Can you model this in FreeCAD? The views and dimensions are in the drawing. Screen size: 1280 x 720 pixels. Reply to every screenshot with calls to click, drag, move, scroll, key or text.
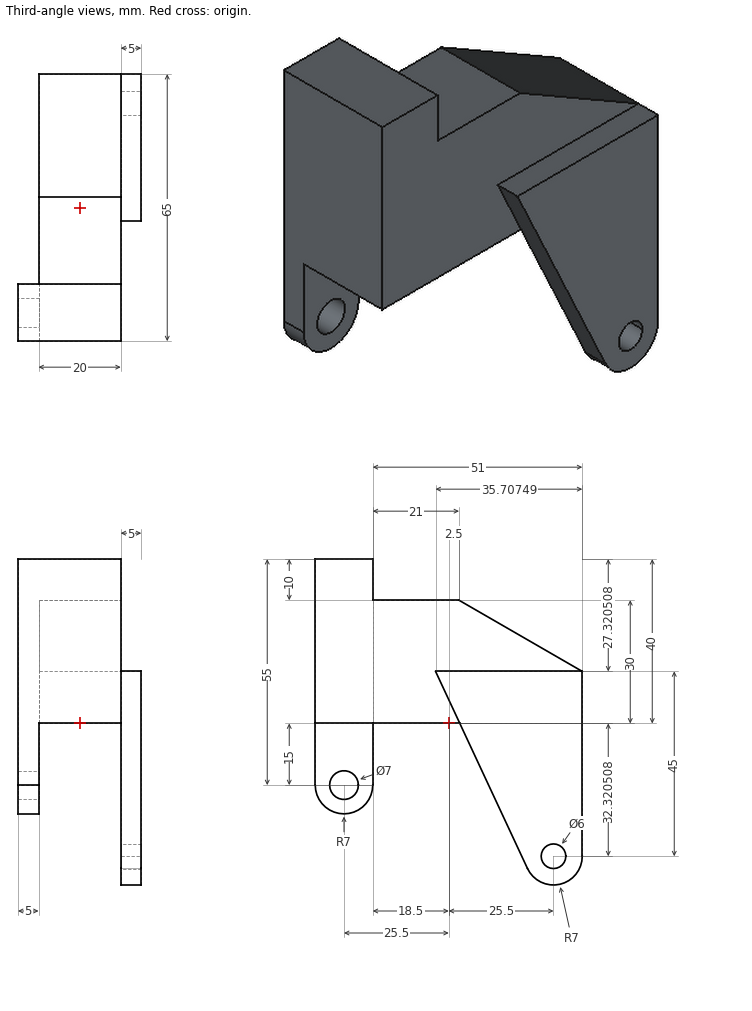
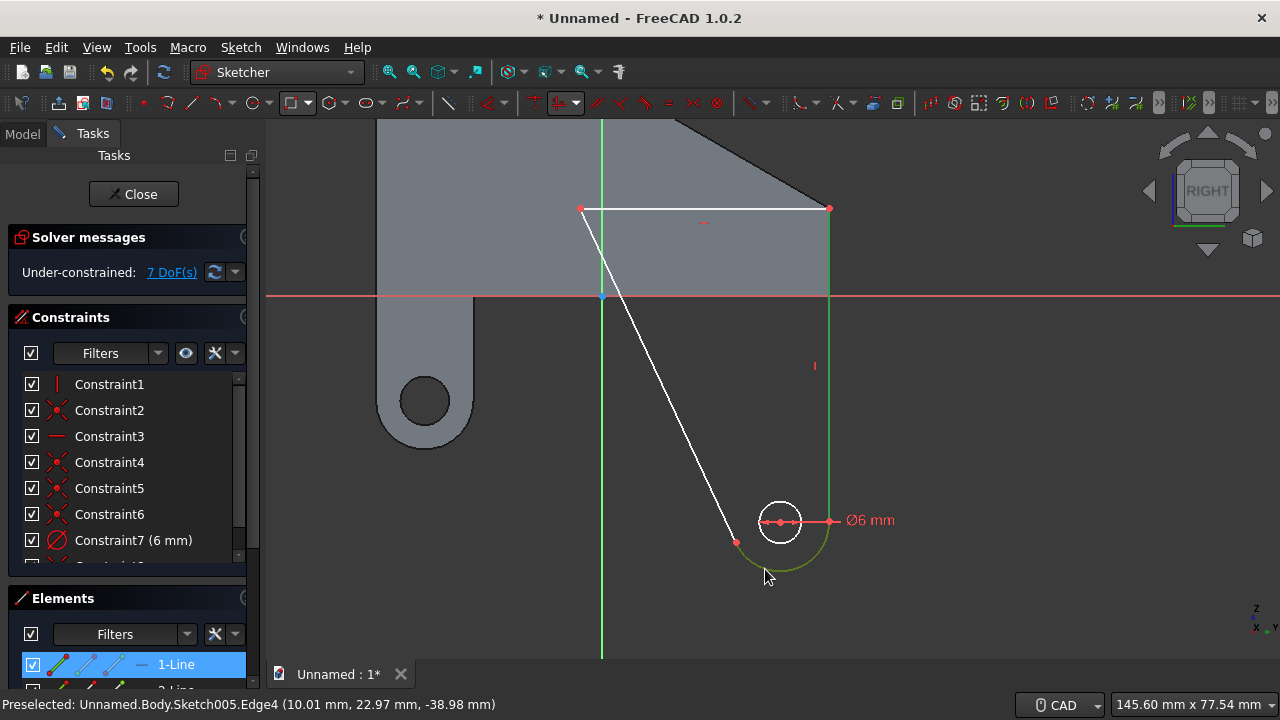
key(t)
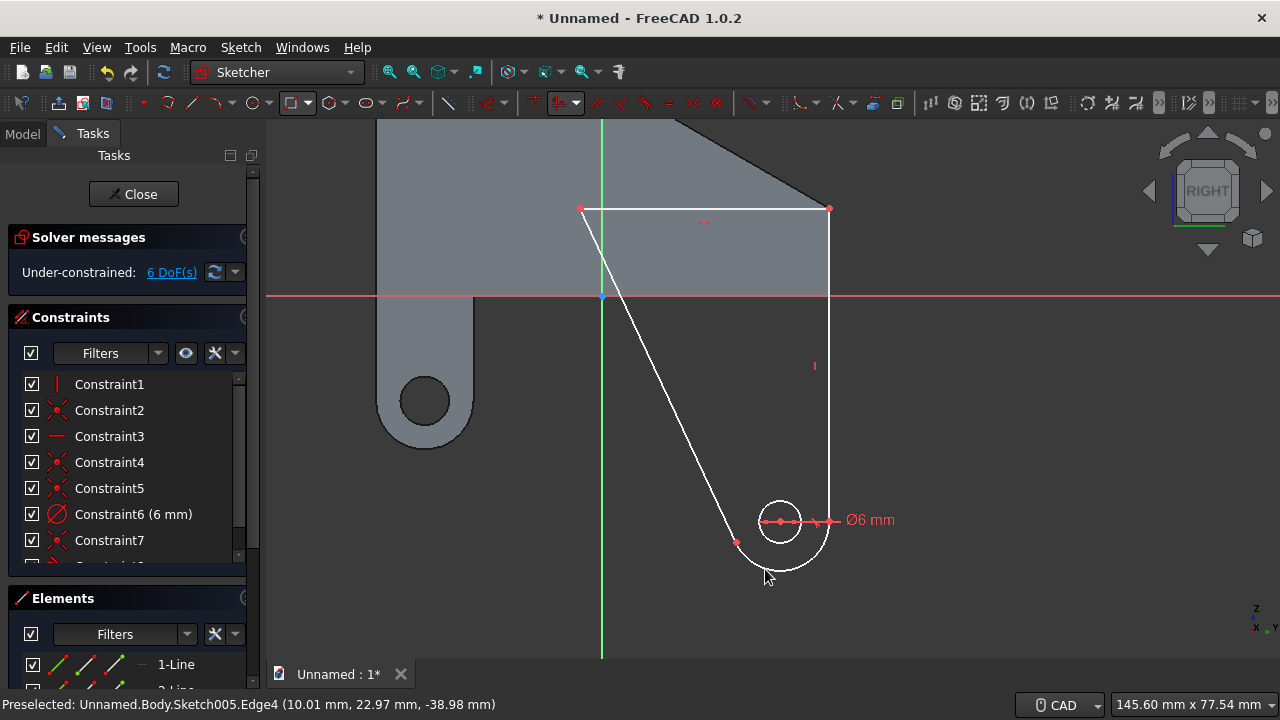
click(627, 309)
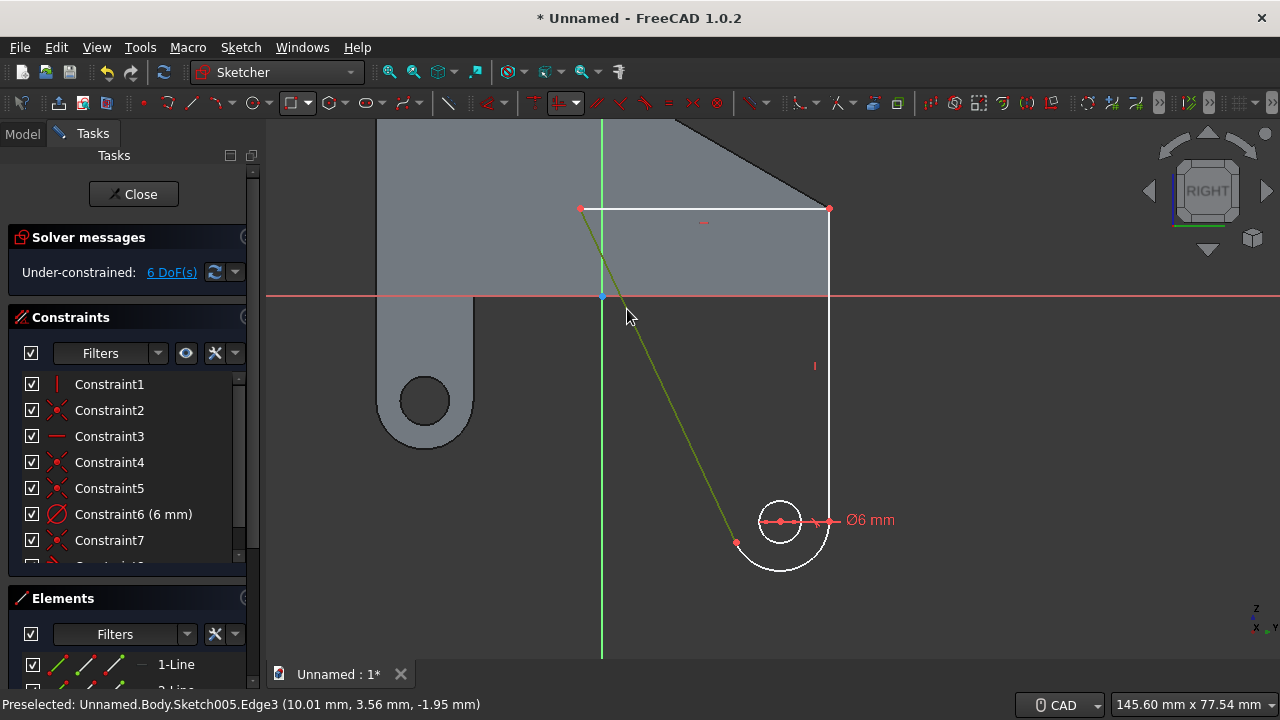
click(765, 568)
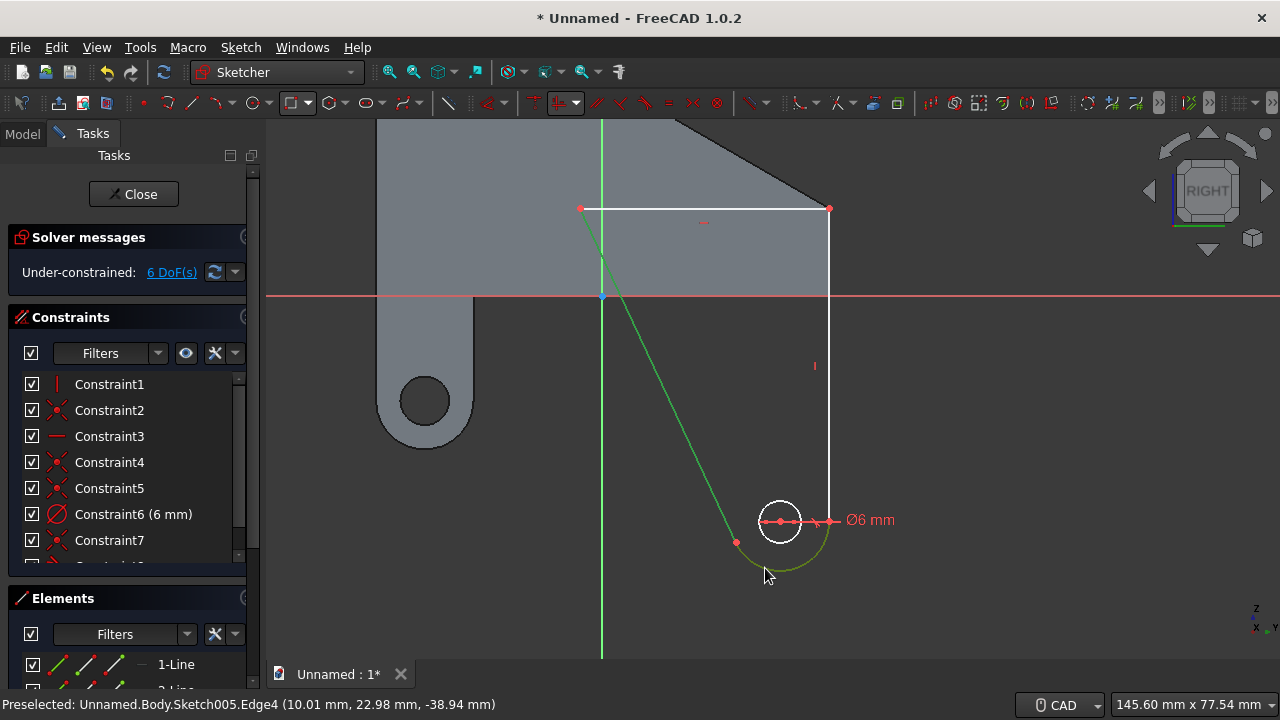
key(t)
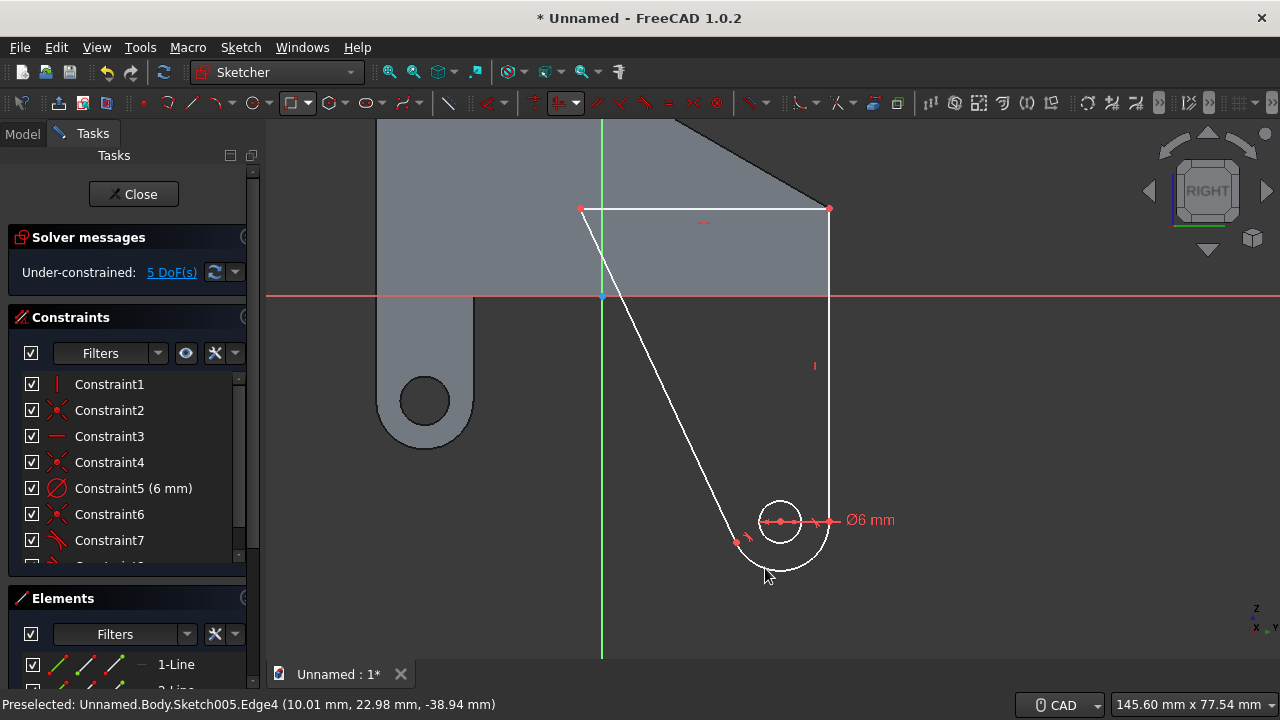
key(d)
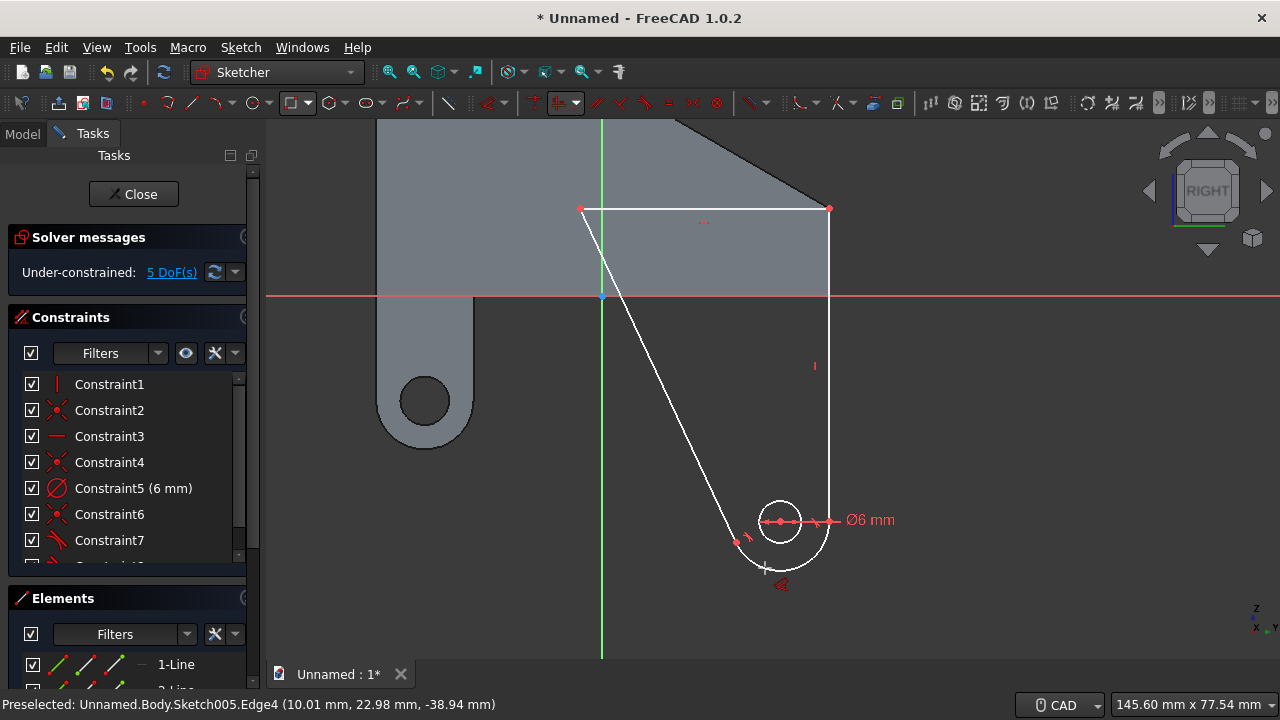
click(765, 568)
click(755, 598)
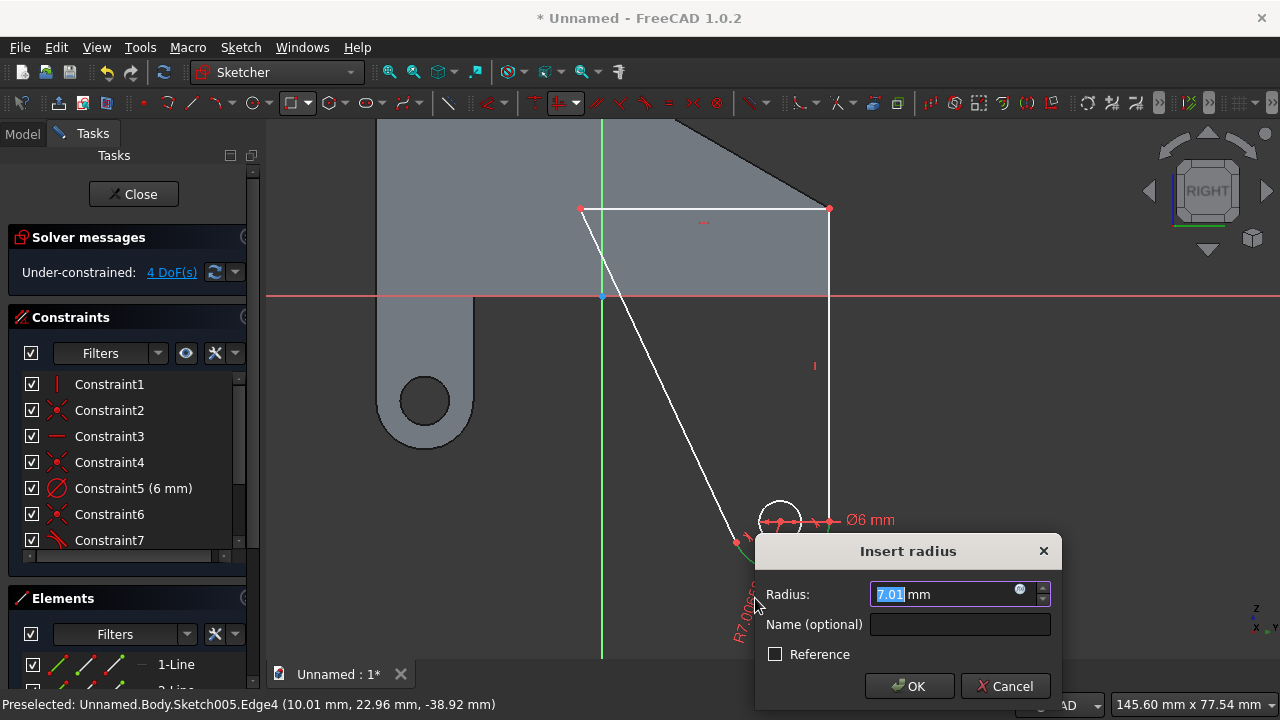
text(7)
key(Return)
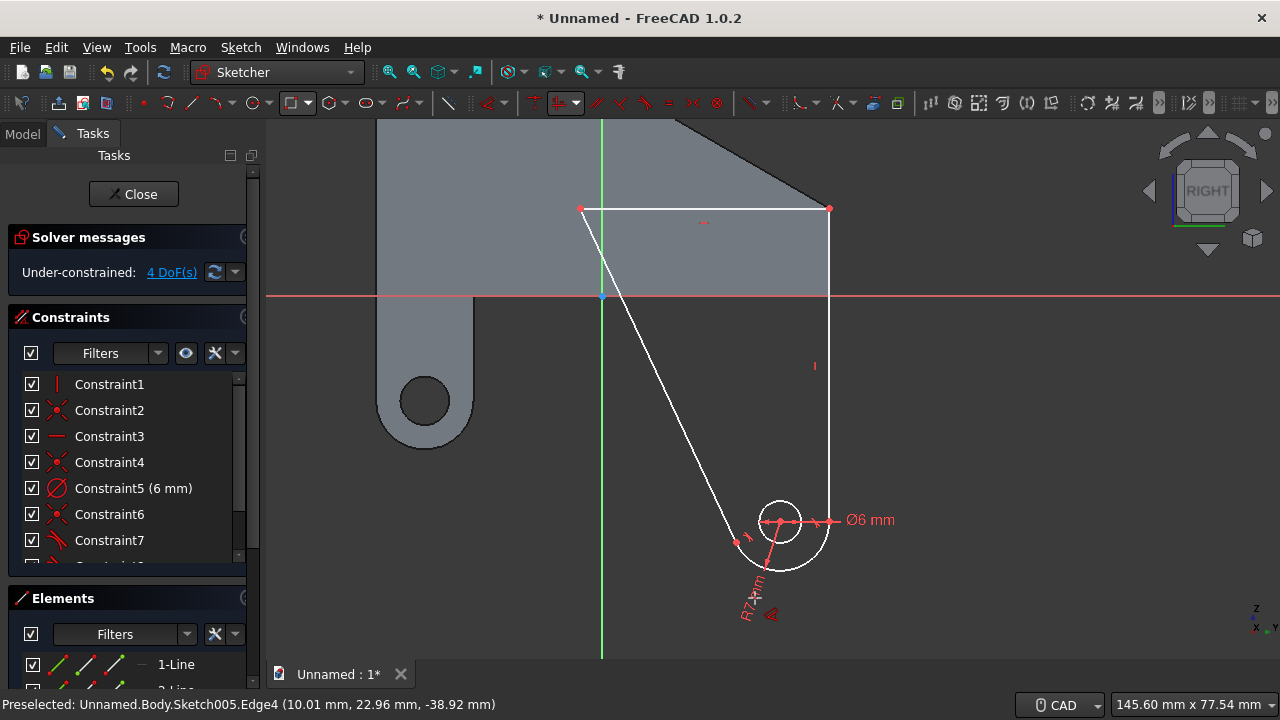
click(829, 428)
click(863, 366)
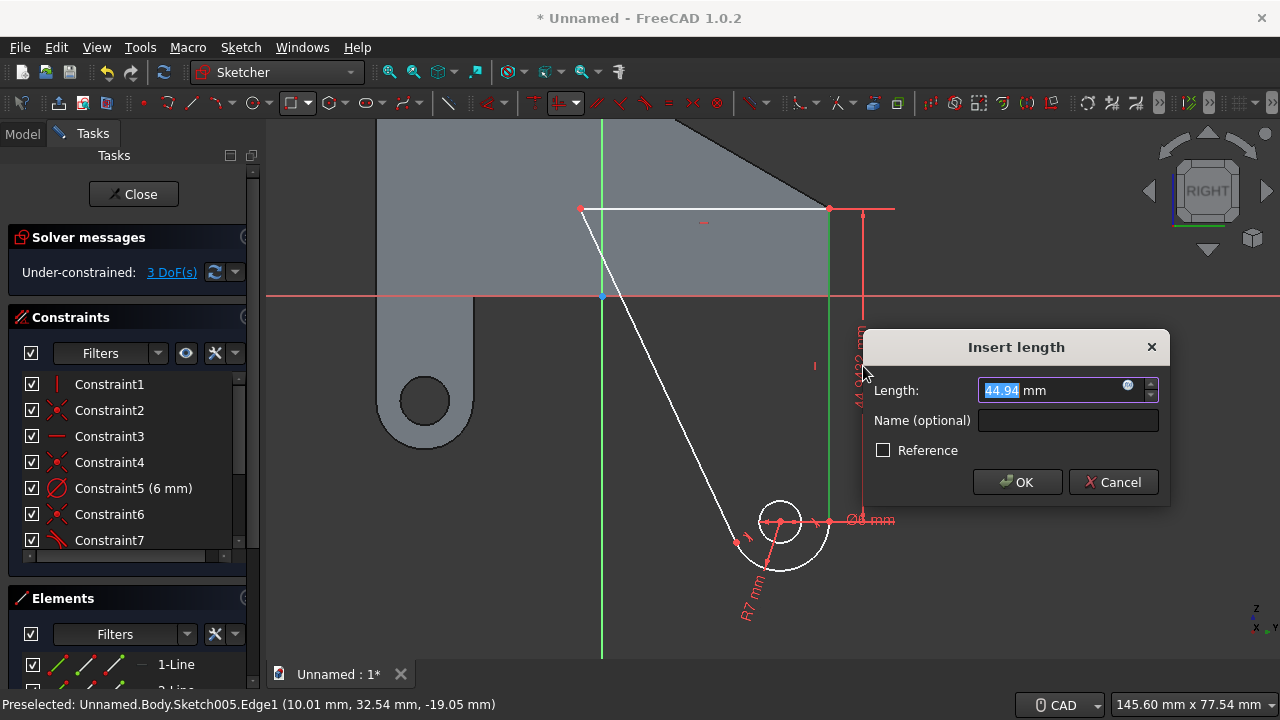
text(45)
key(Return)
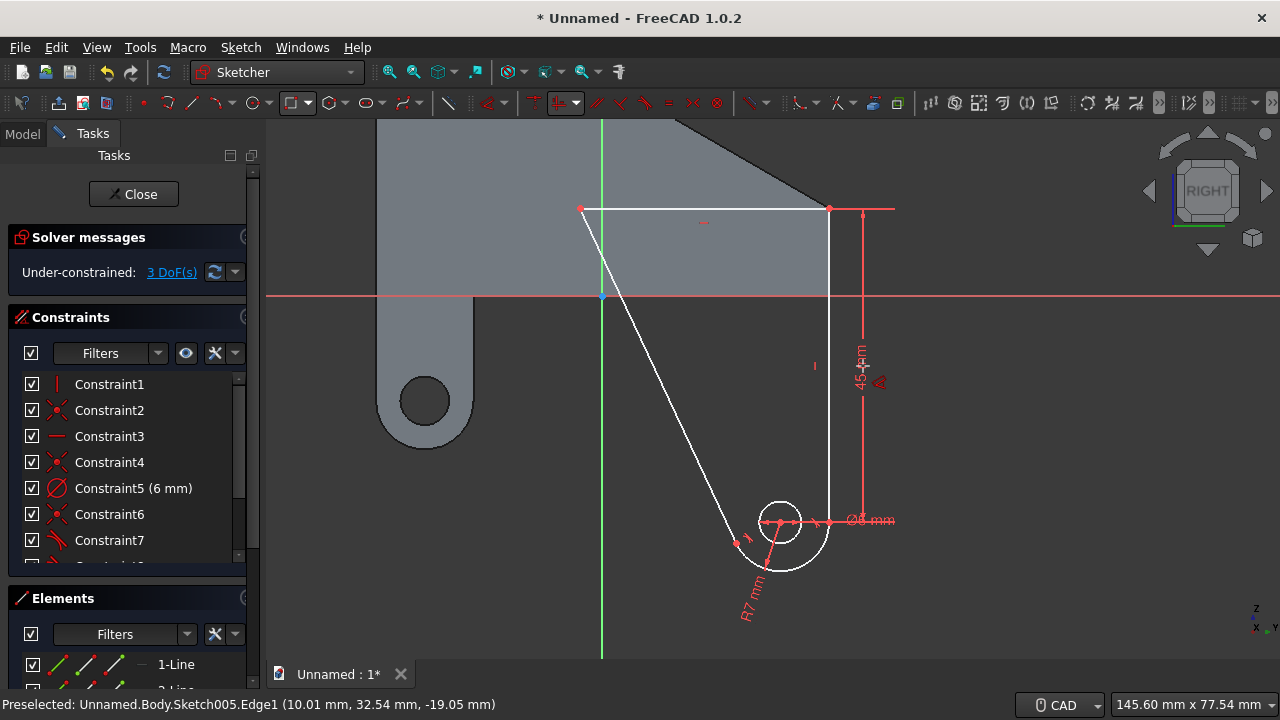
click(780, 522)
click(691, 556)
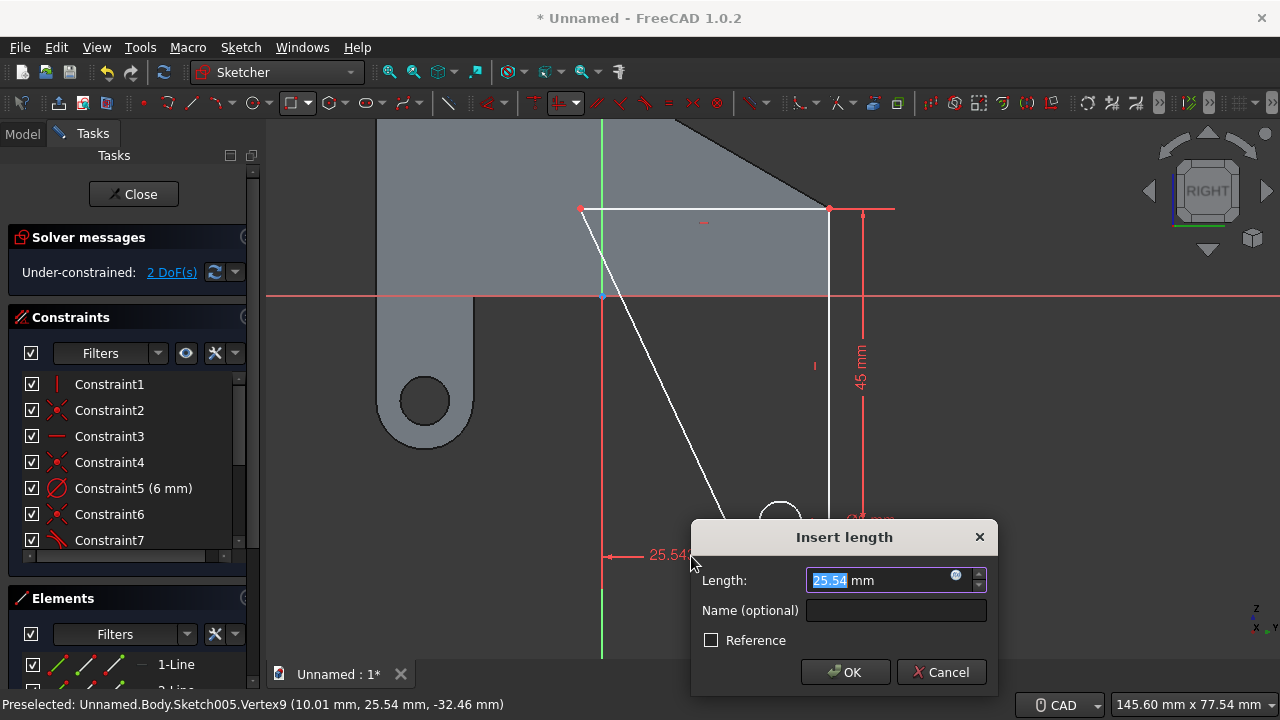
text(25.5)
key(Return)